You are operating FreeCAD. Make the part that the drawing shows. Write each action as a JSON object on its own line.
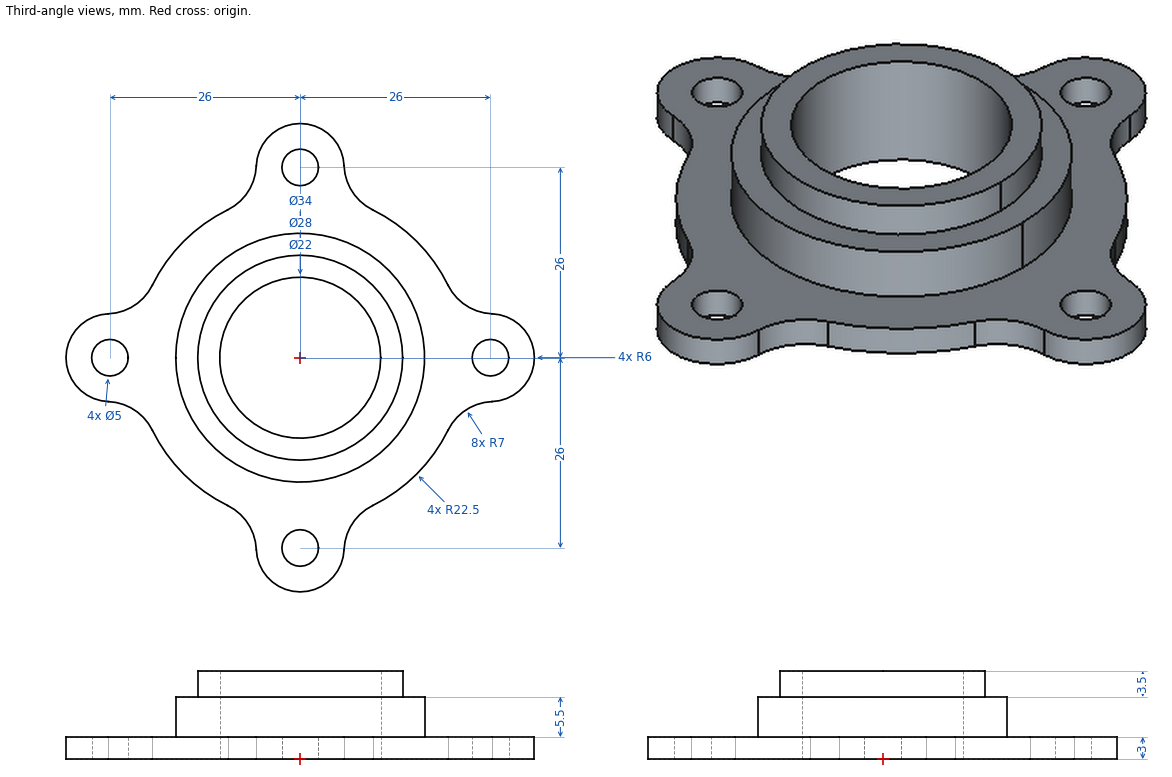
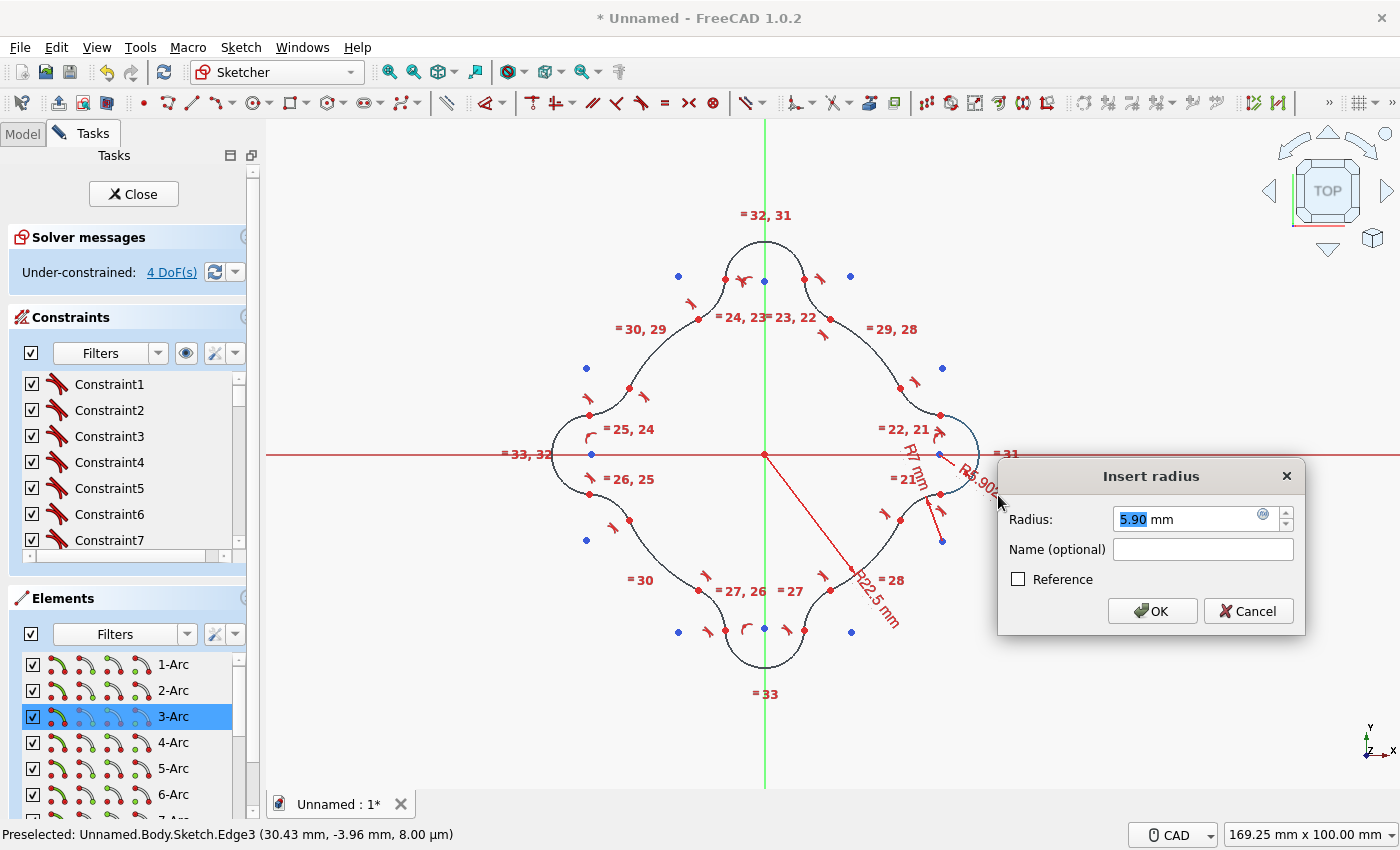
{"action": "type", "text": "6"}
{"action": "key", "text": "Return"}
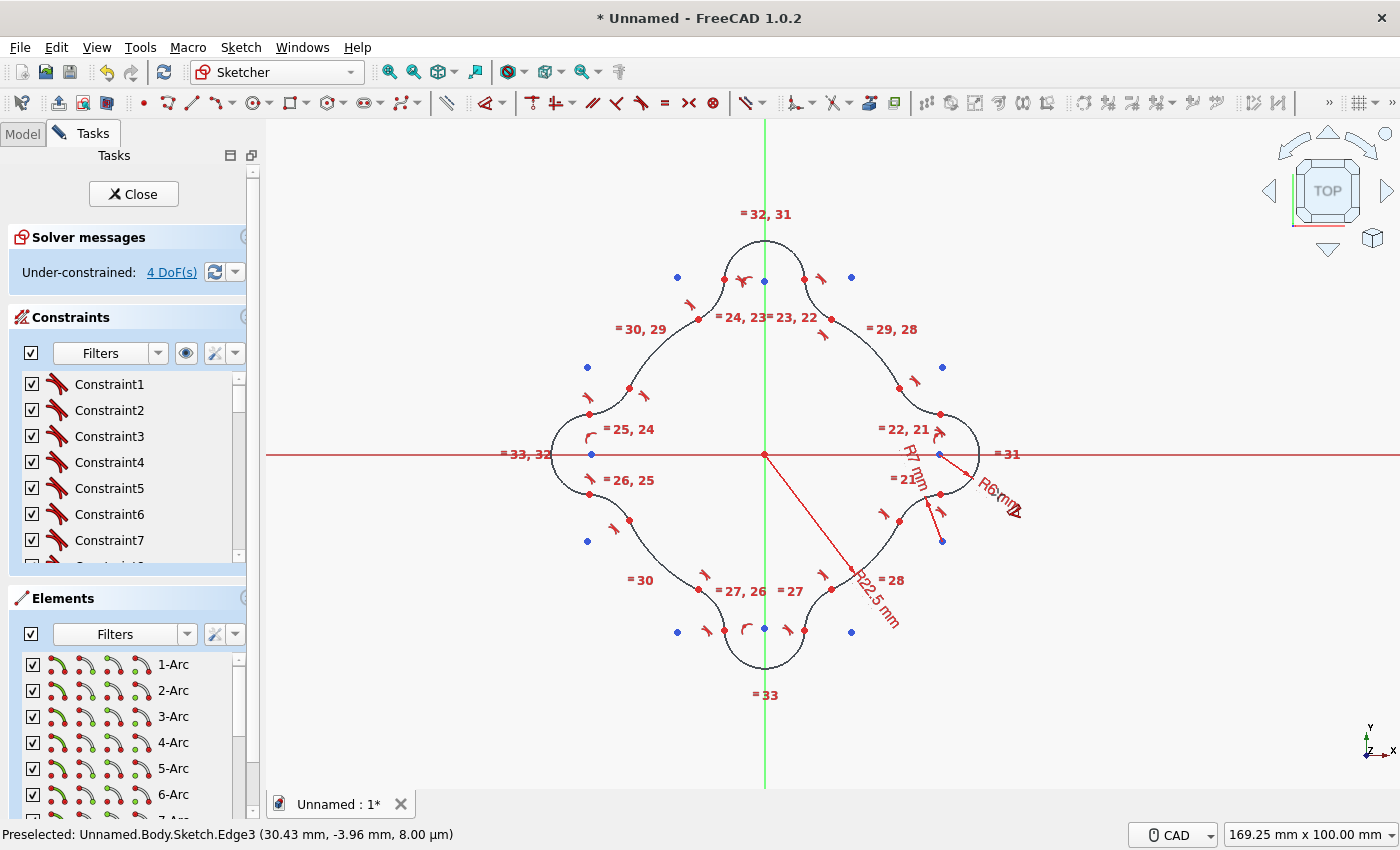
{"action": "left_click", "coordinate": [939, 455]}
{"action": "left_click", "coordinate": [852, 489]}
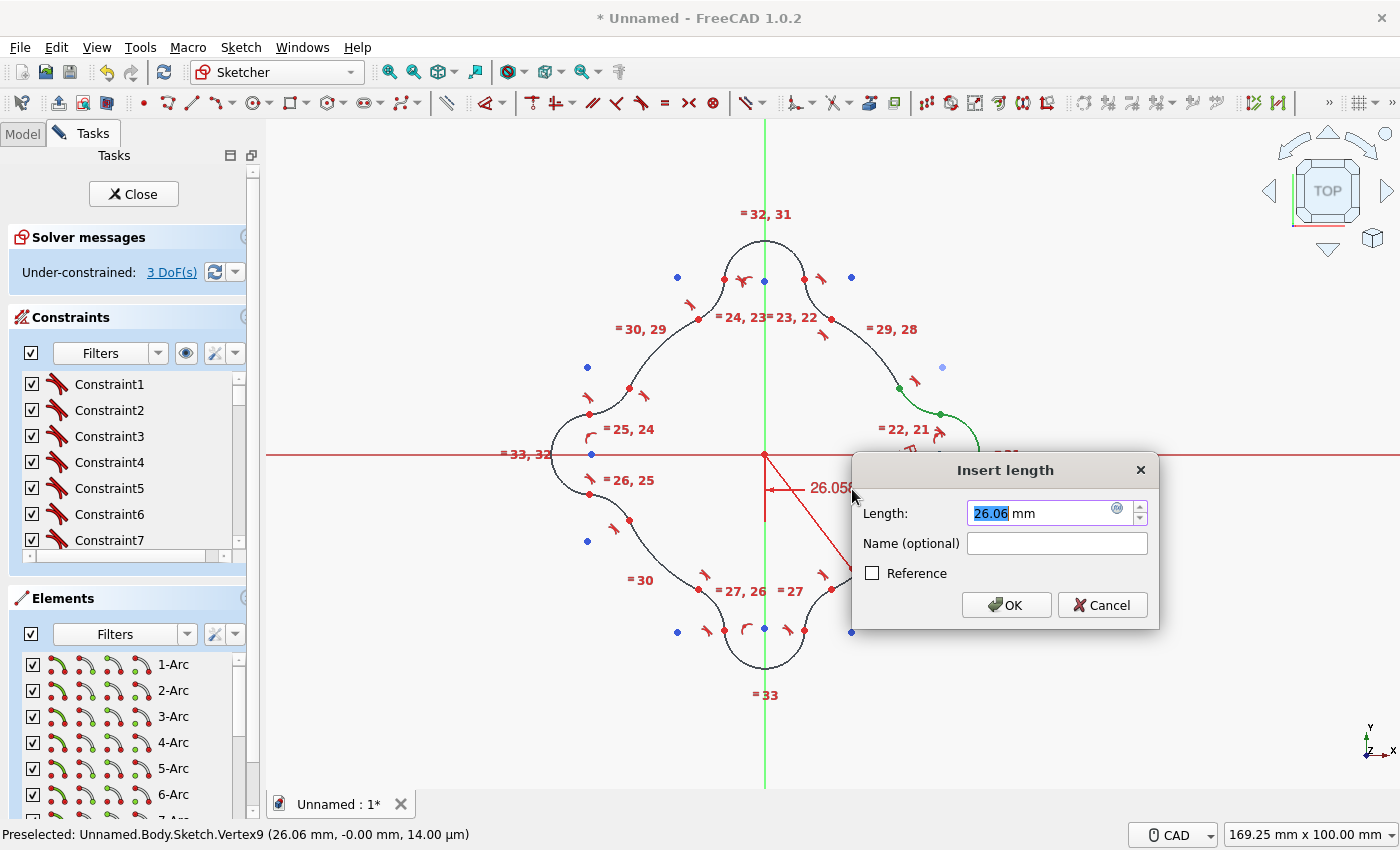
{"action": "type", "text": "26"}
{"action": "key", "text": "Return"}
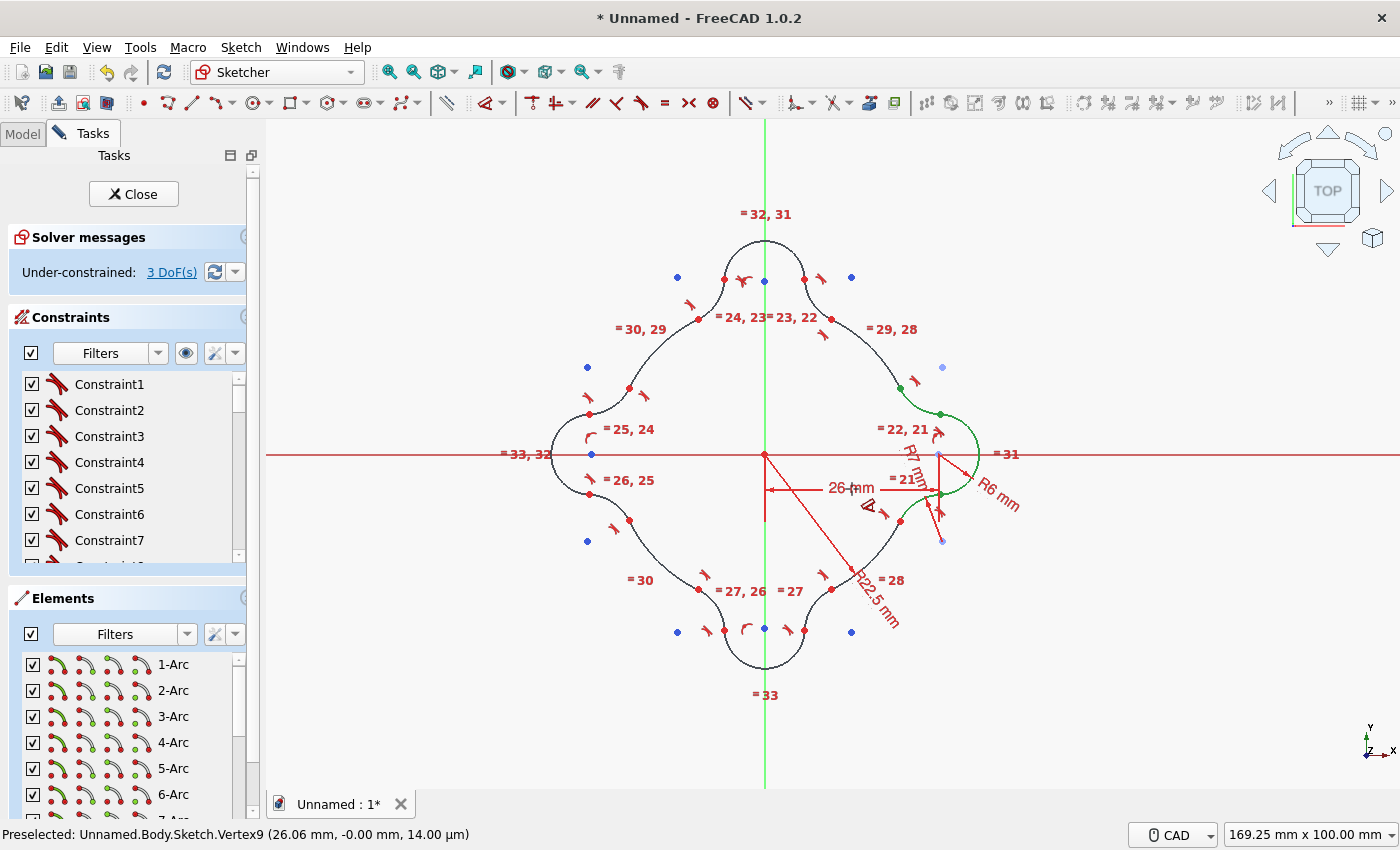
{"action": "left_click", "coordinate": [765, 281]}
{"action": "left_click", "coordinate": [799, 368]}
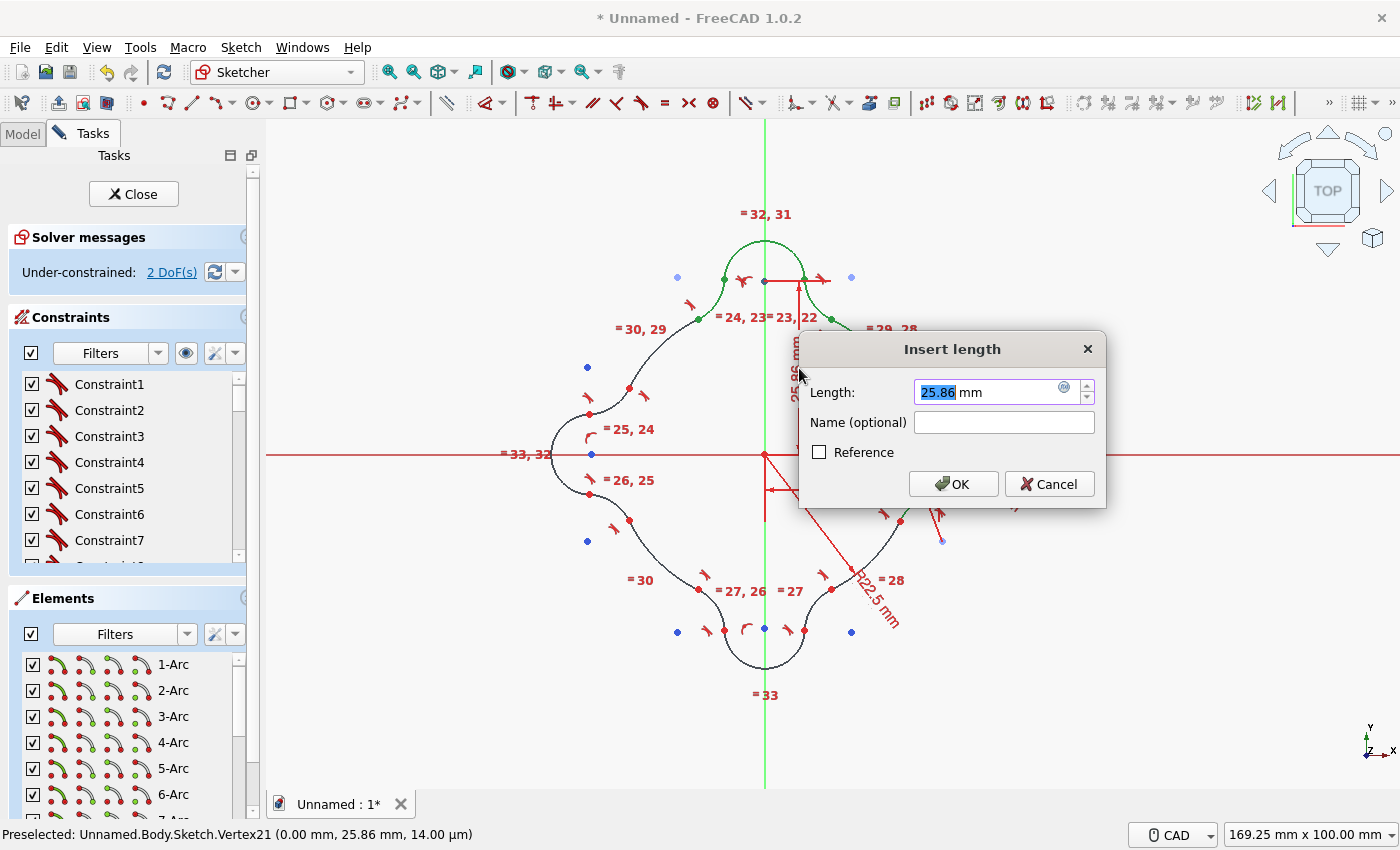
{"action": "type", "text": "26"}
{"action": "key", "text": "Return"}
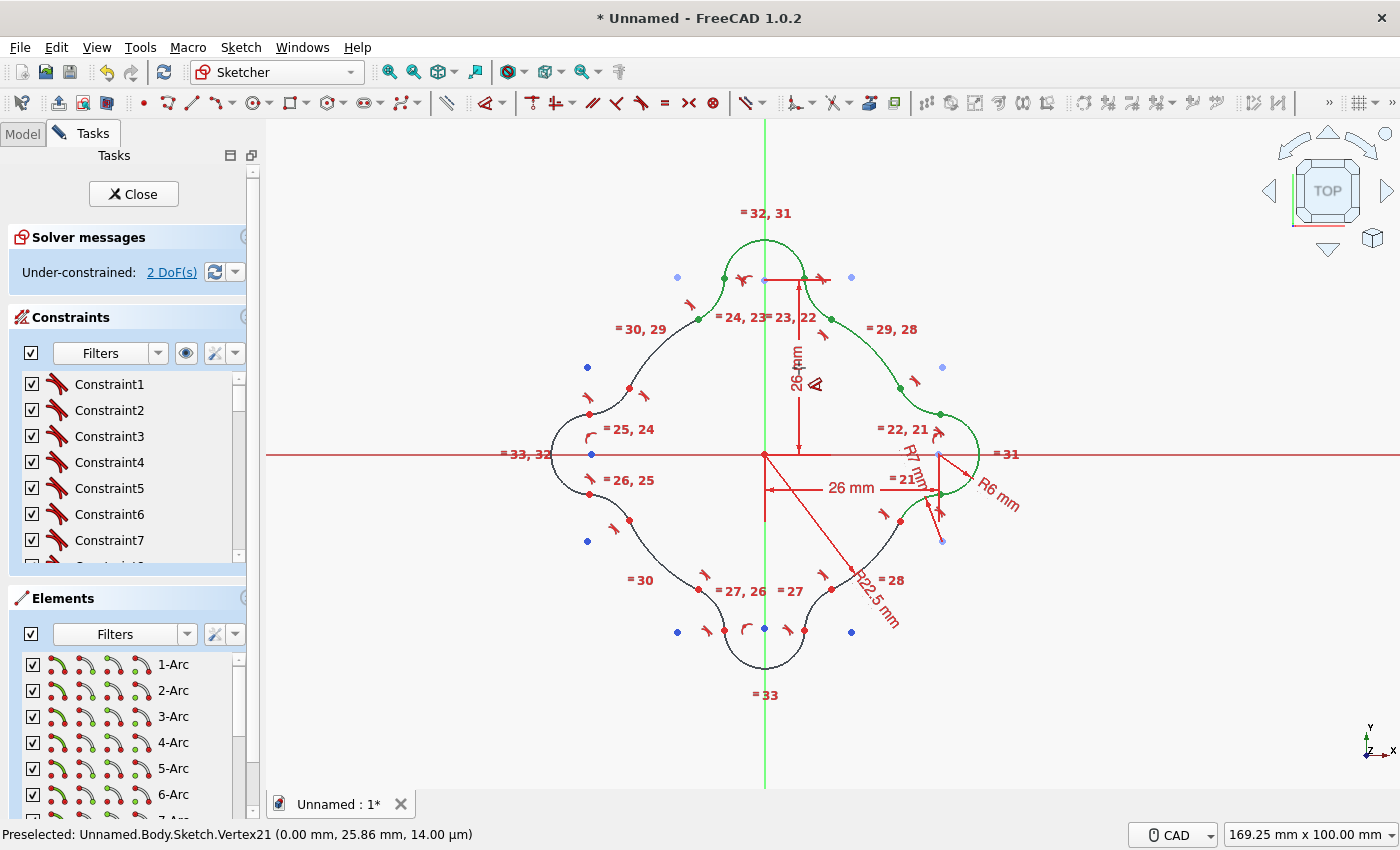
{"action": "left_click", "coordinate": [591, 455]}
{"action": "left_click", "coordinate": [678, 489]}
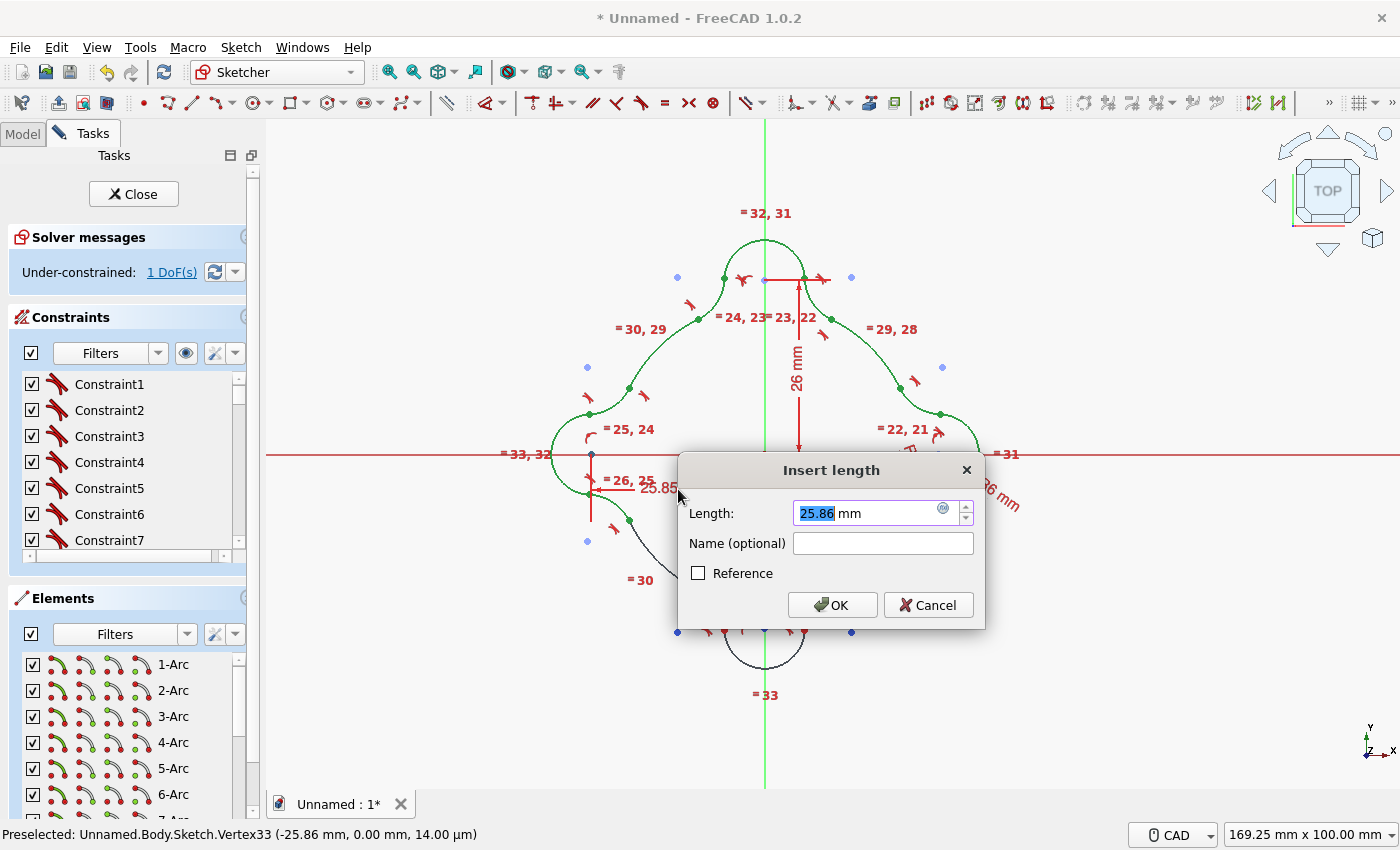
{"action": "type", "text": "26"}
{"action": "key", "text": "Return"}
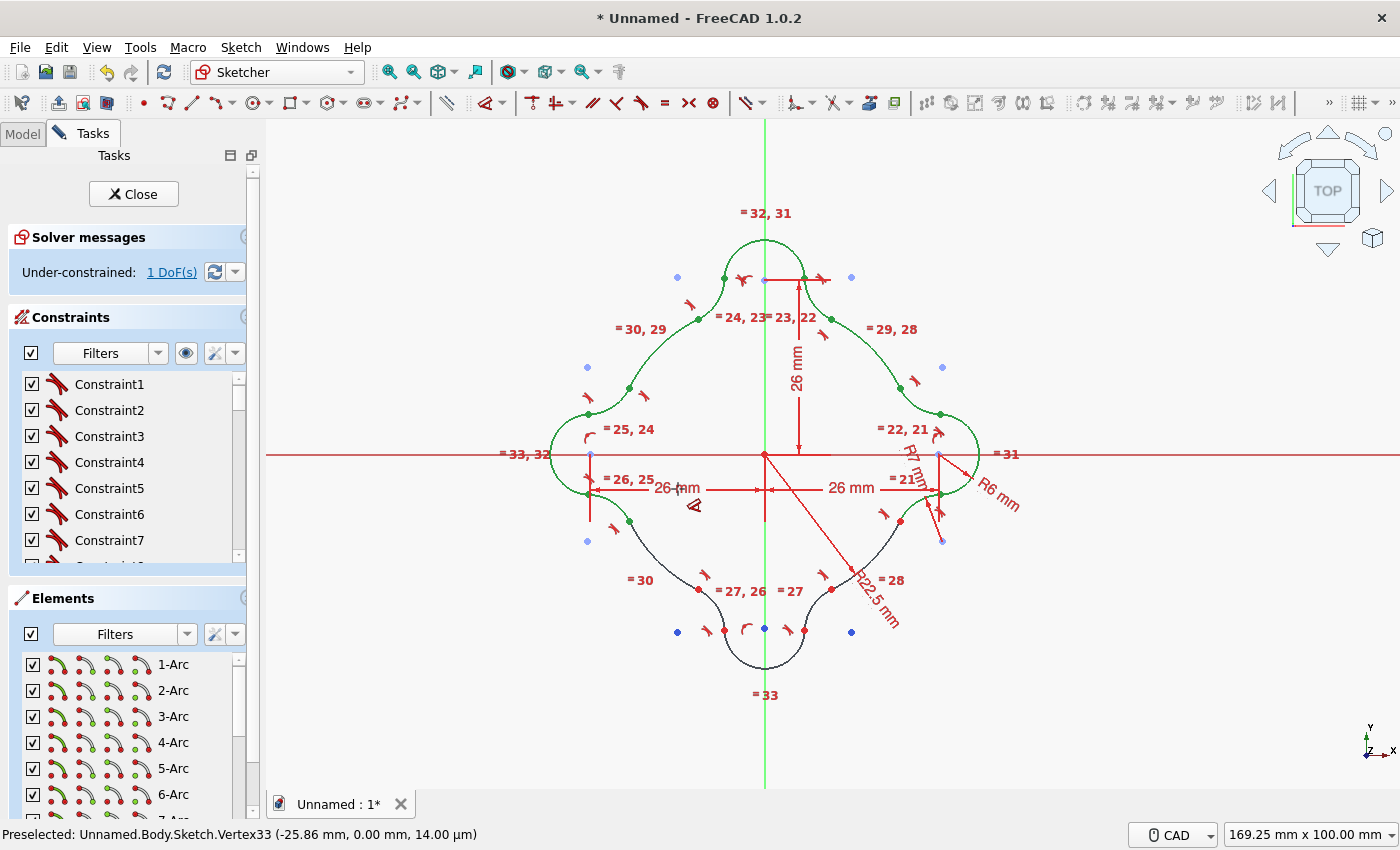
{"action": "left_click", "coordinate": [765, 629]}
{"action": "left_click", "coordinate": [799, 542]}